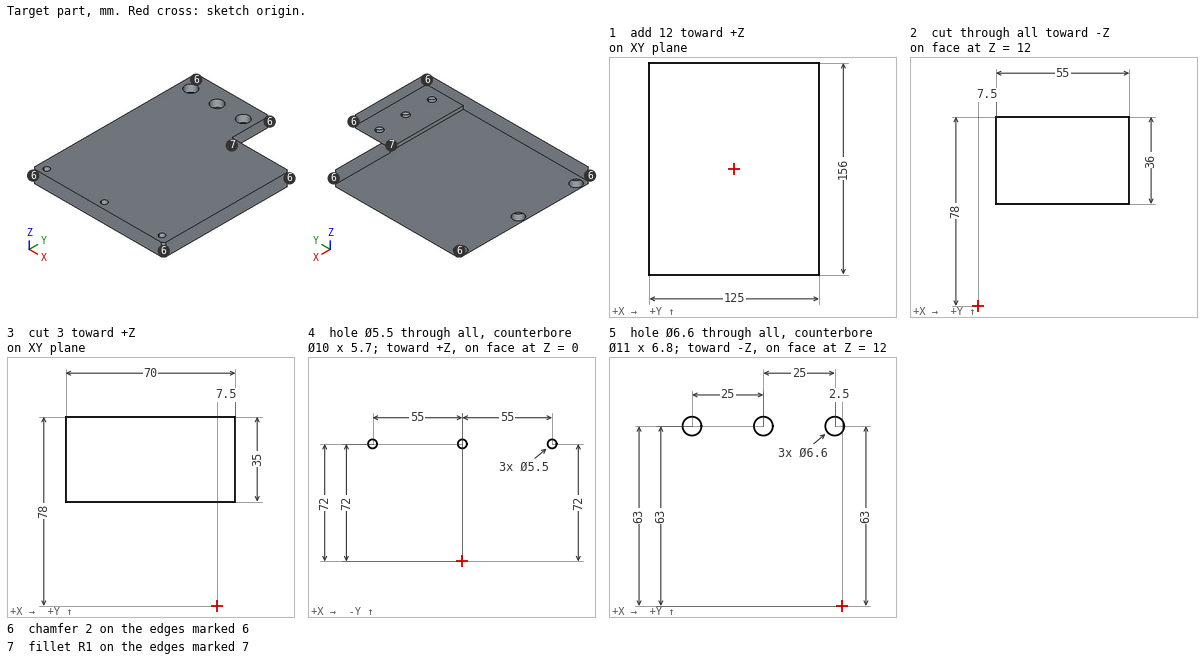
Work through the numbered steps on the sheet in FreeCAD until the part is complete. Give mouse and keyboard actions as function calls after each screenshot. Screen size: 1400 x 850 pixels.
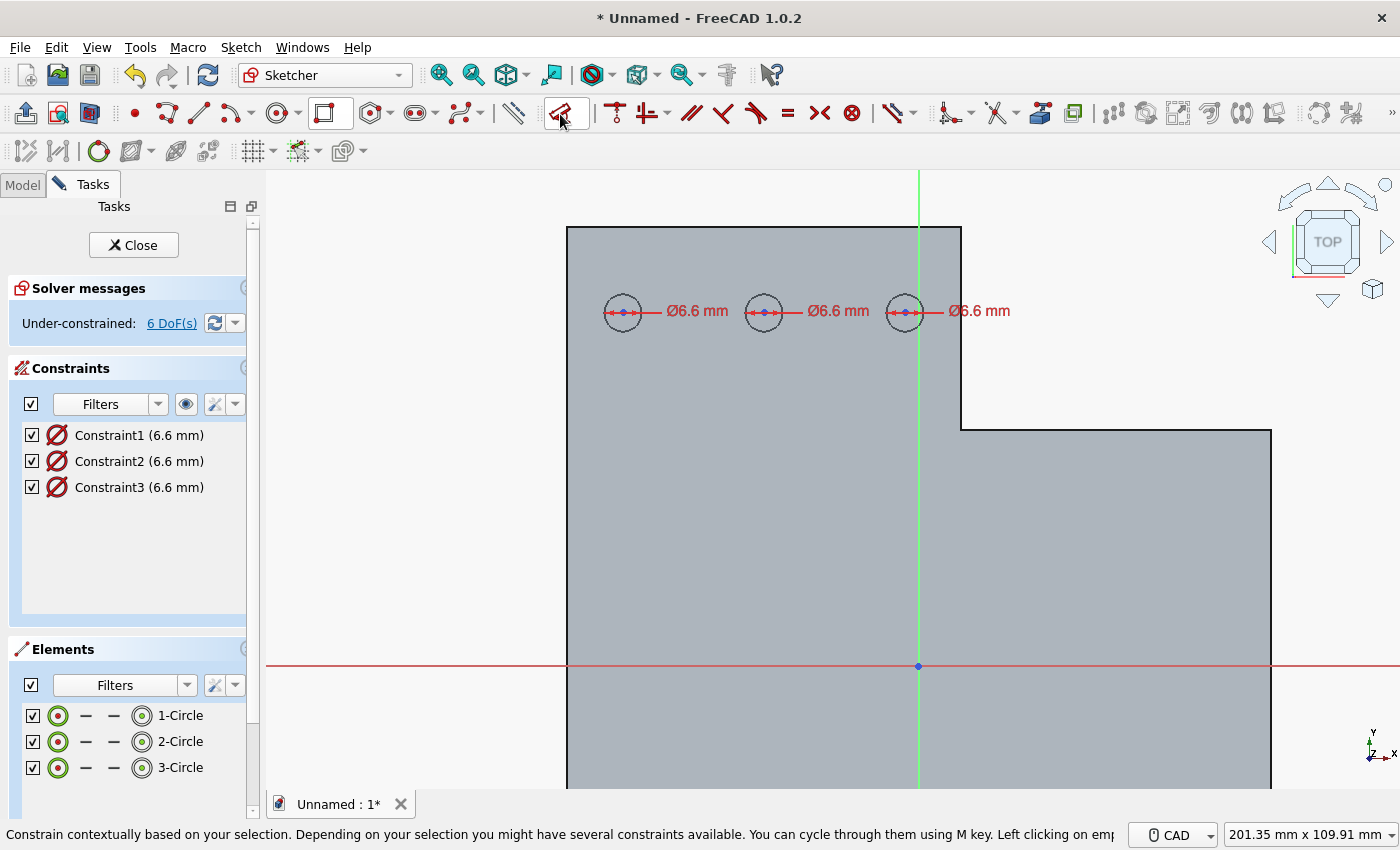
click(905, 313)
click(953, 490)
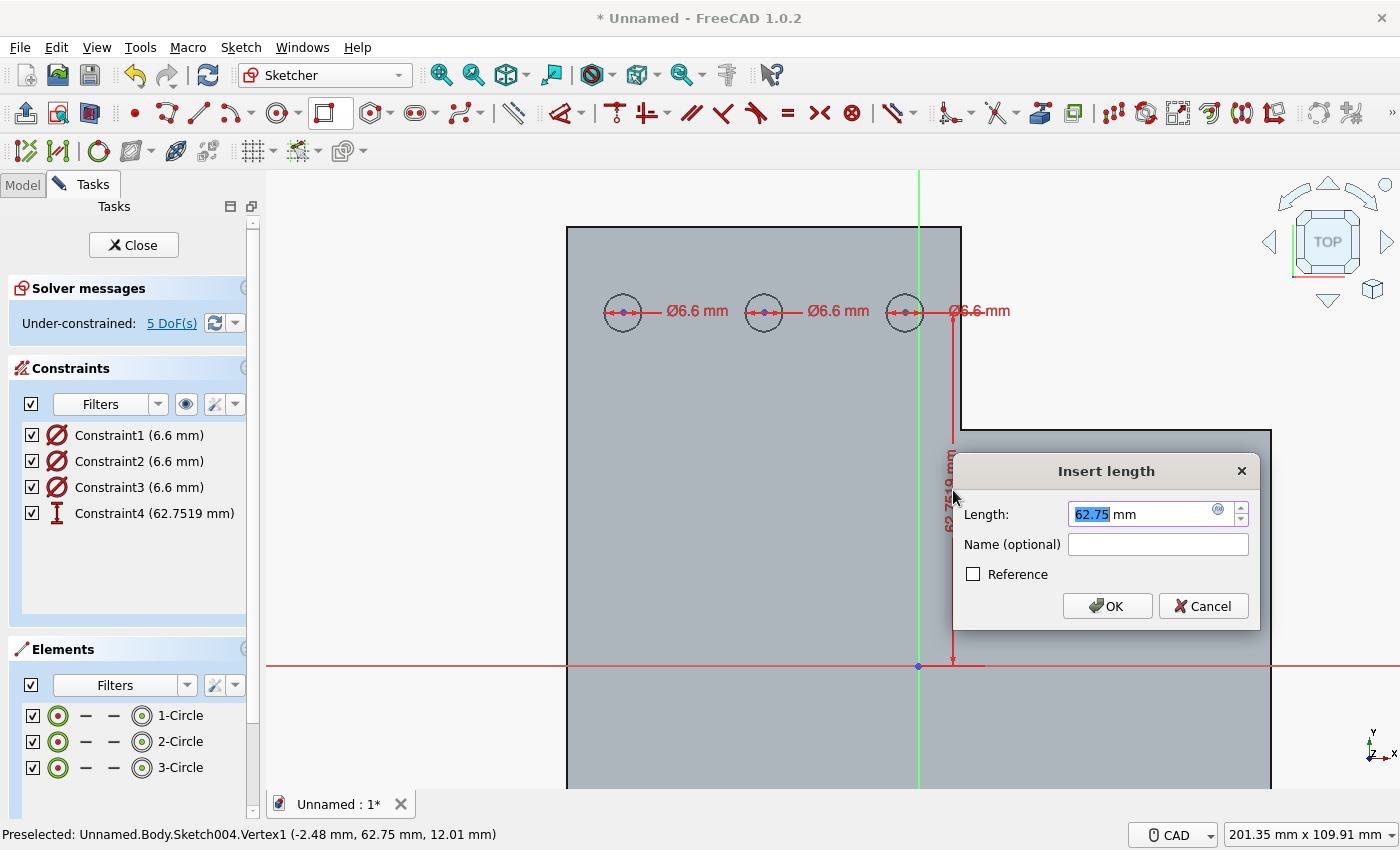
text(63)
key(Return)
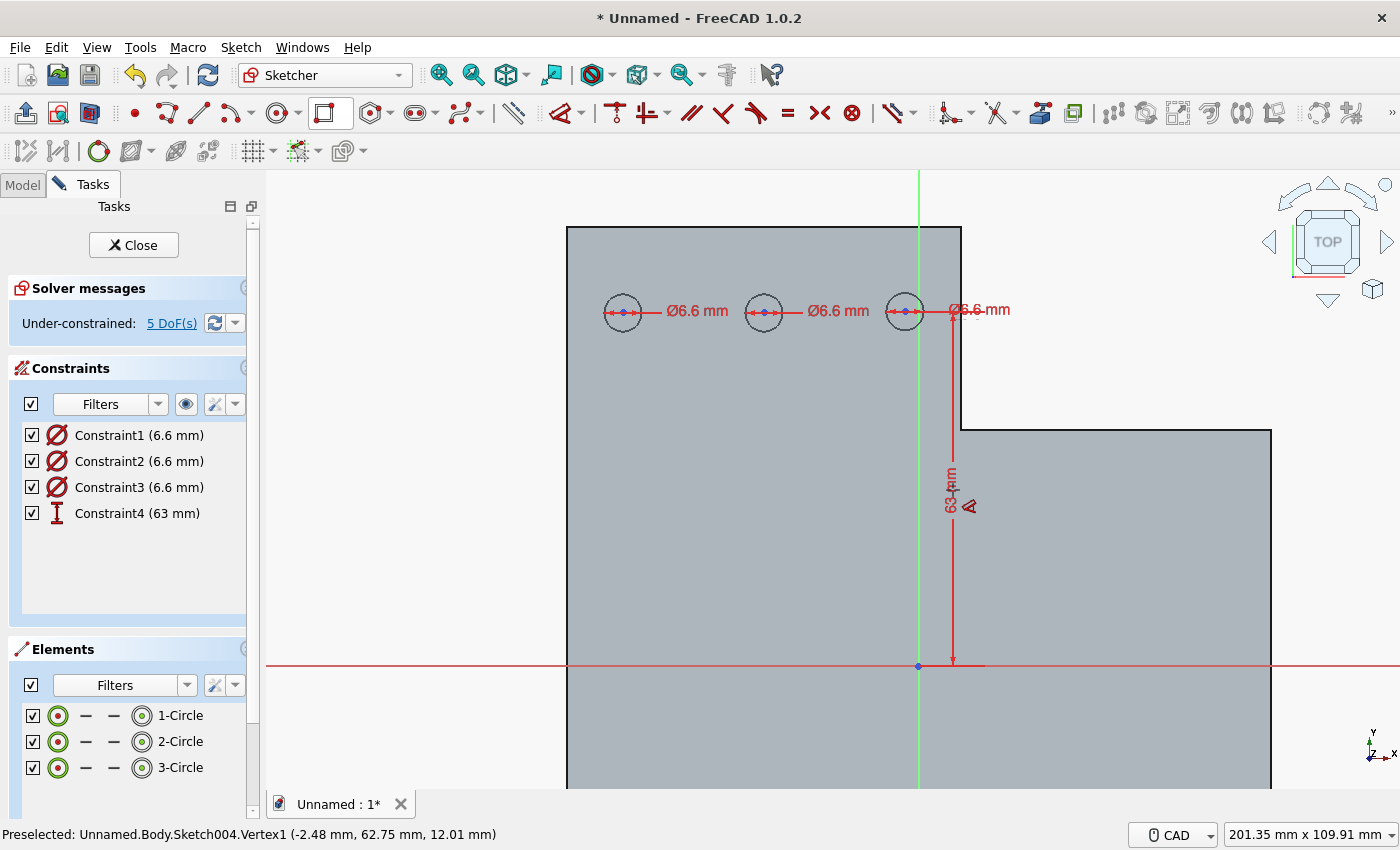
click(764, 313)
click(953, 408)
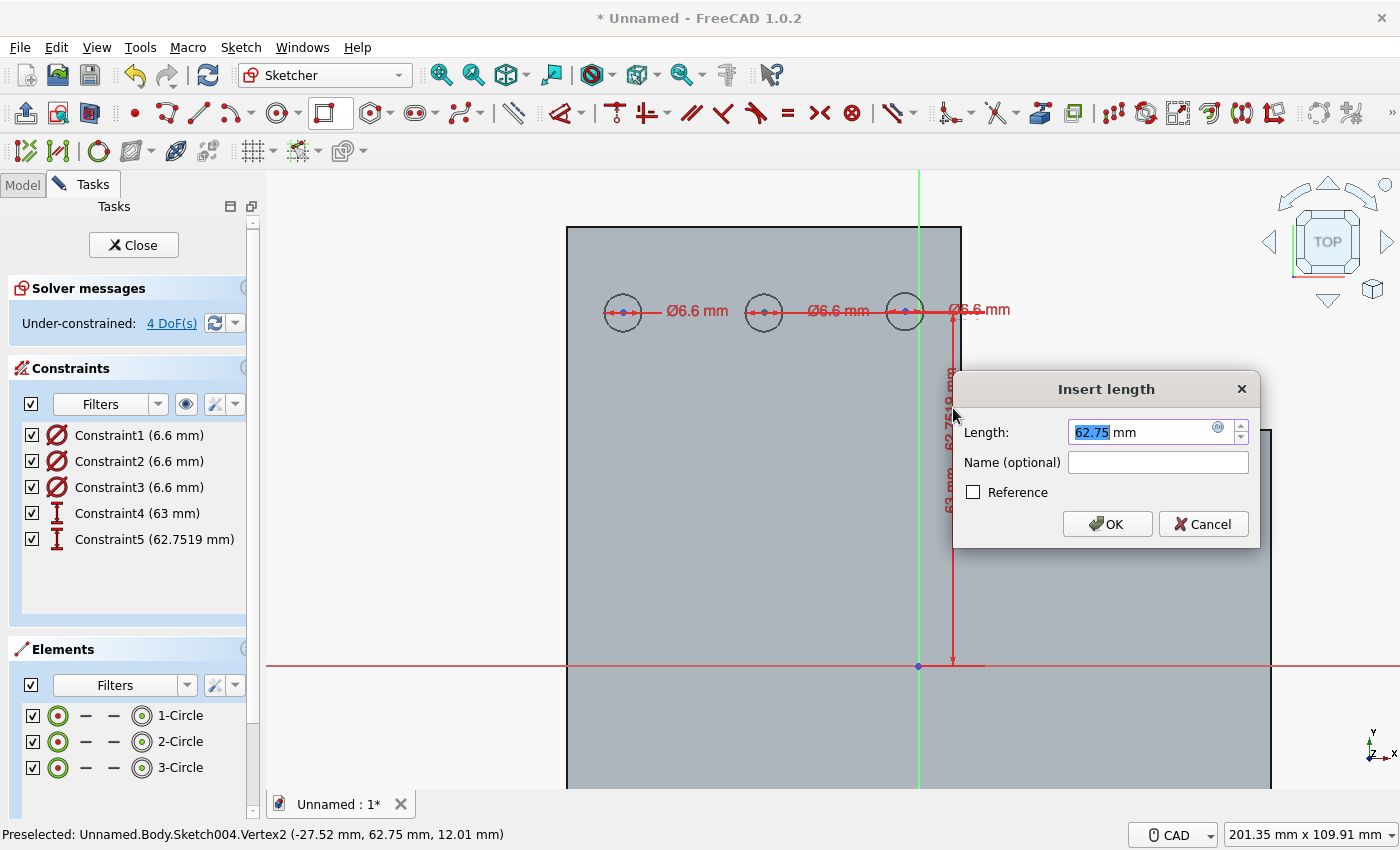
text(63)
key(Return)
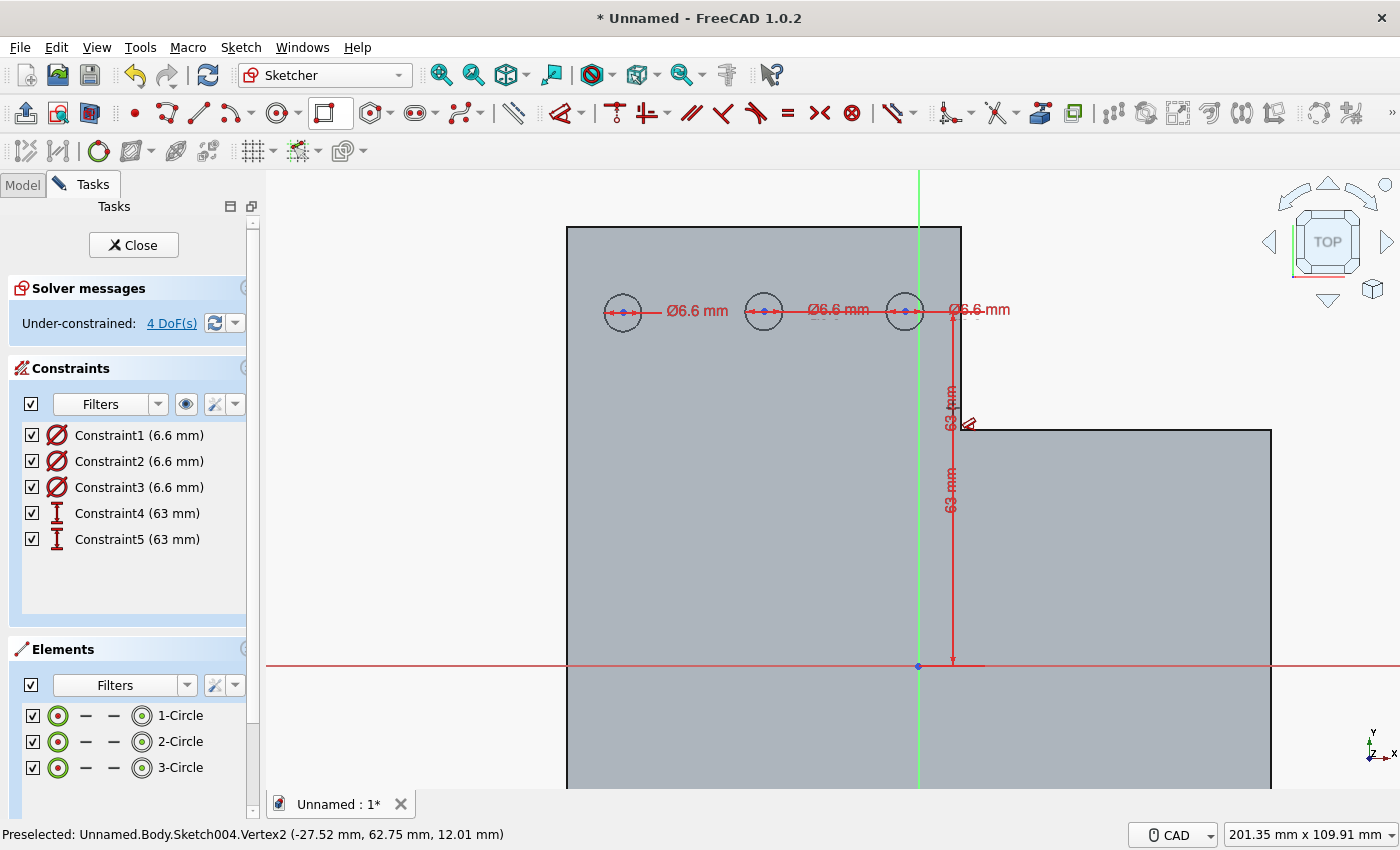
click(623, 313)
click(953, 571)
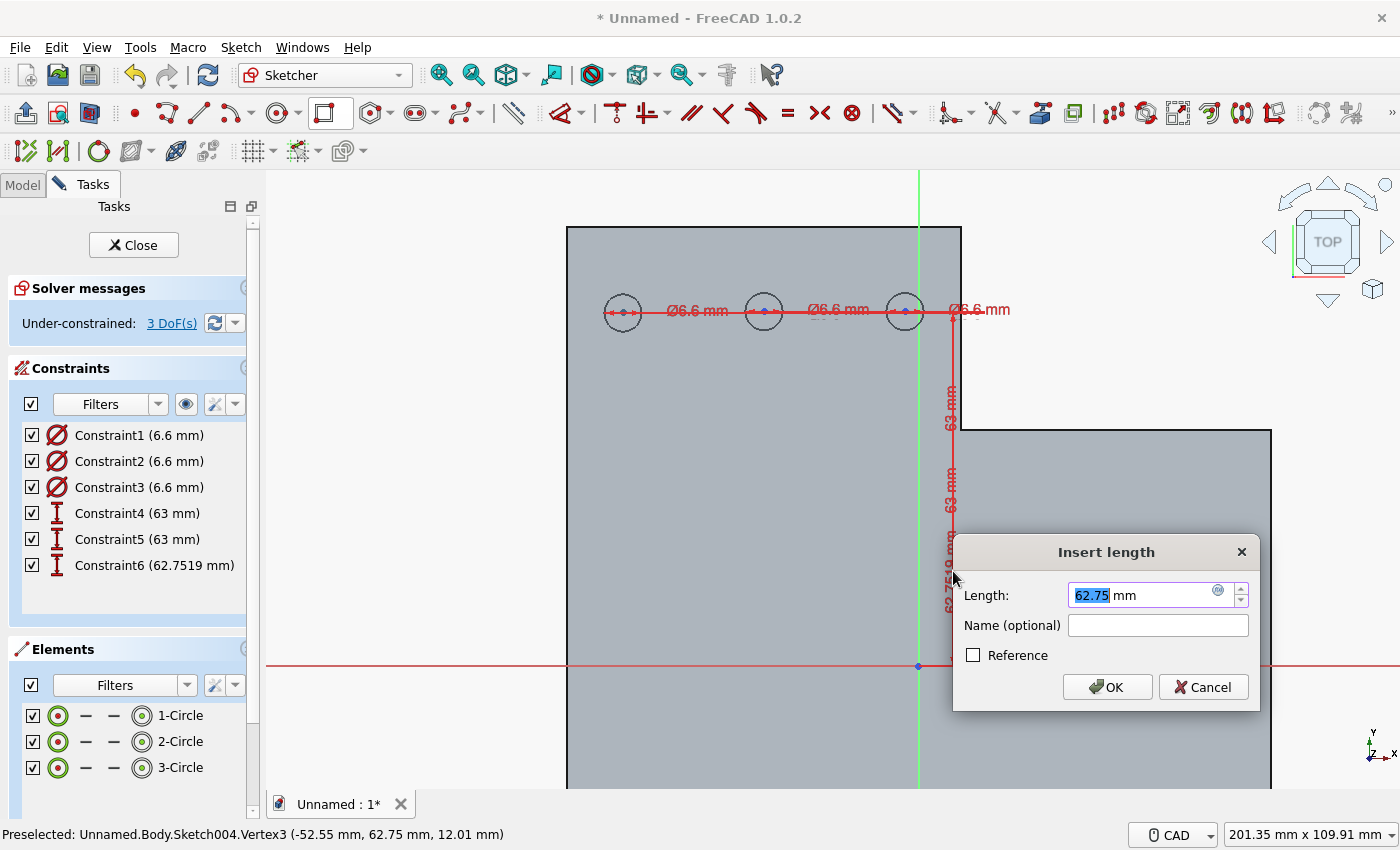
text(63)
key(Return)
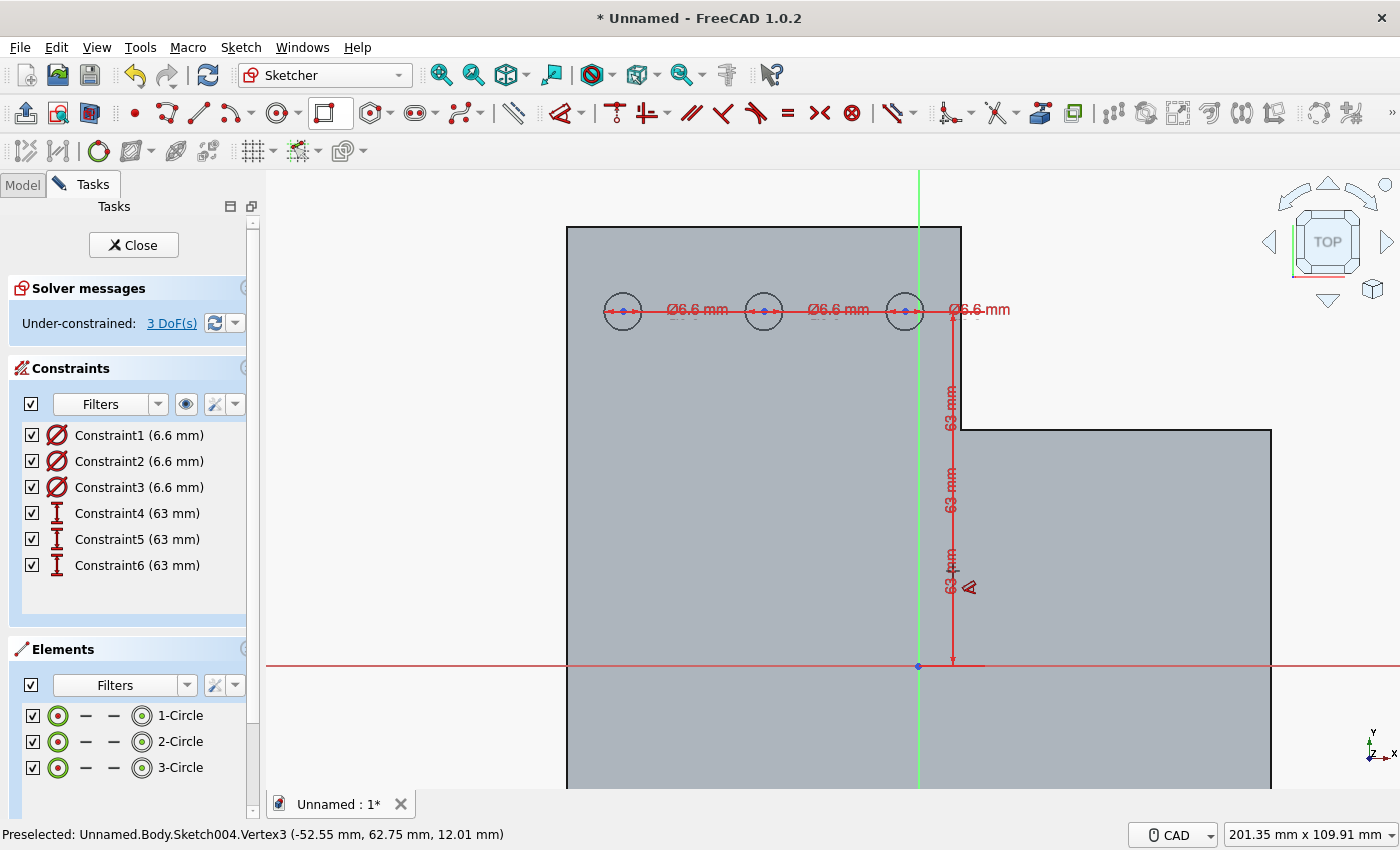
scroll(905, 312, up, 6)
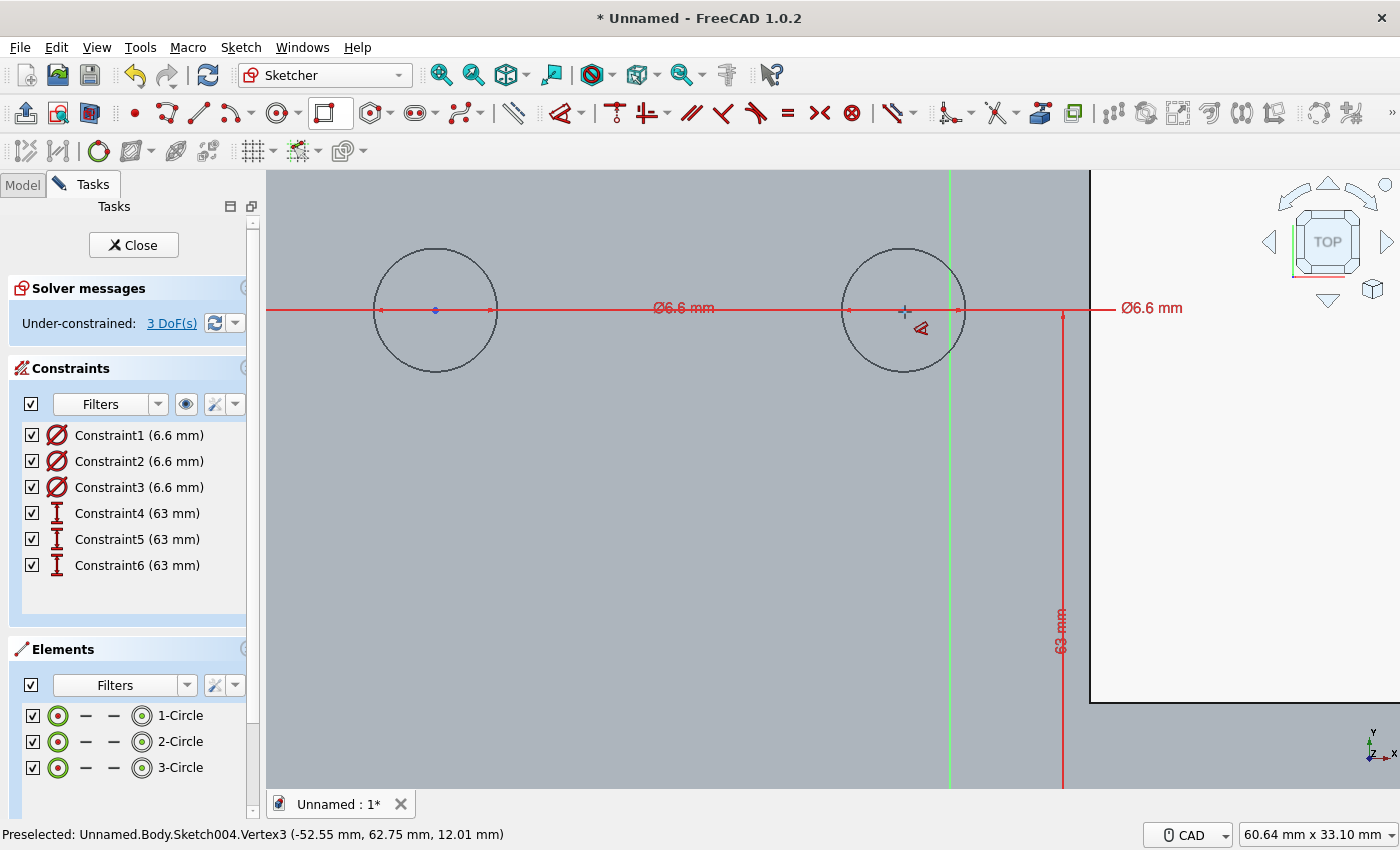
click(904, 310)
click(927, 276)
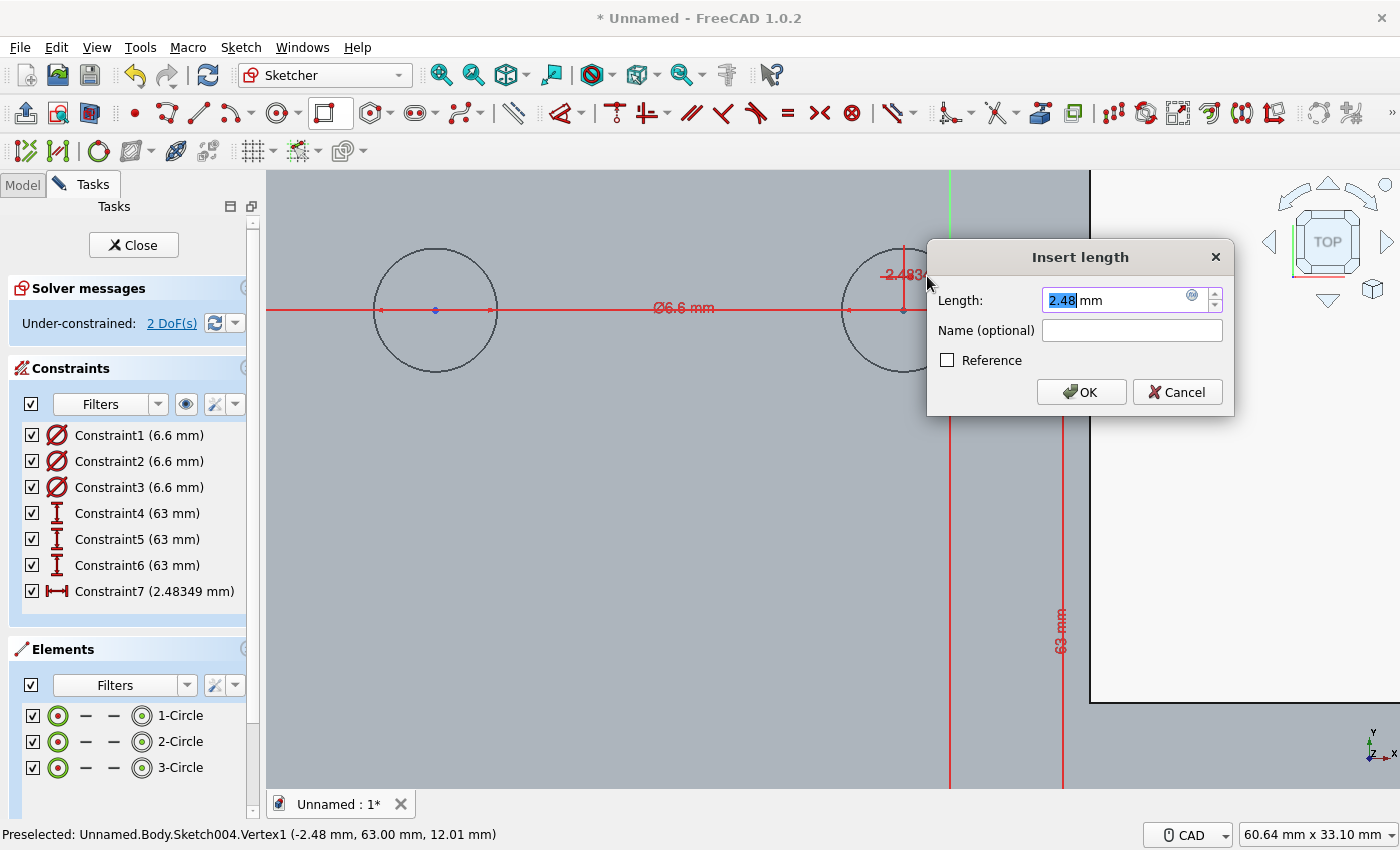
text(2.5)
key(Return)